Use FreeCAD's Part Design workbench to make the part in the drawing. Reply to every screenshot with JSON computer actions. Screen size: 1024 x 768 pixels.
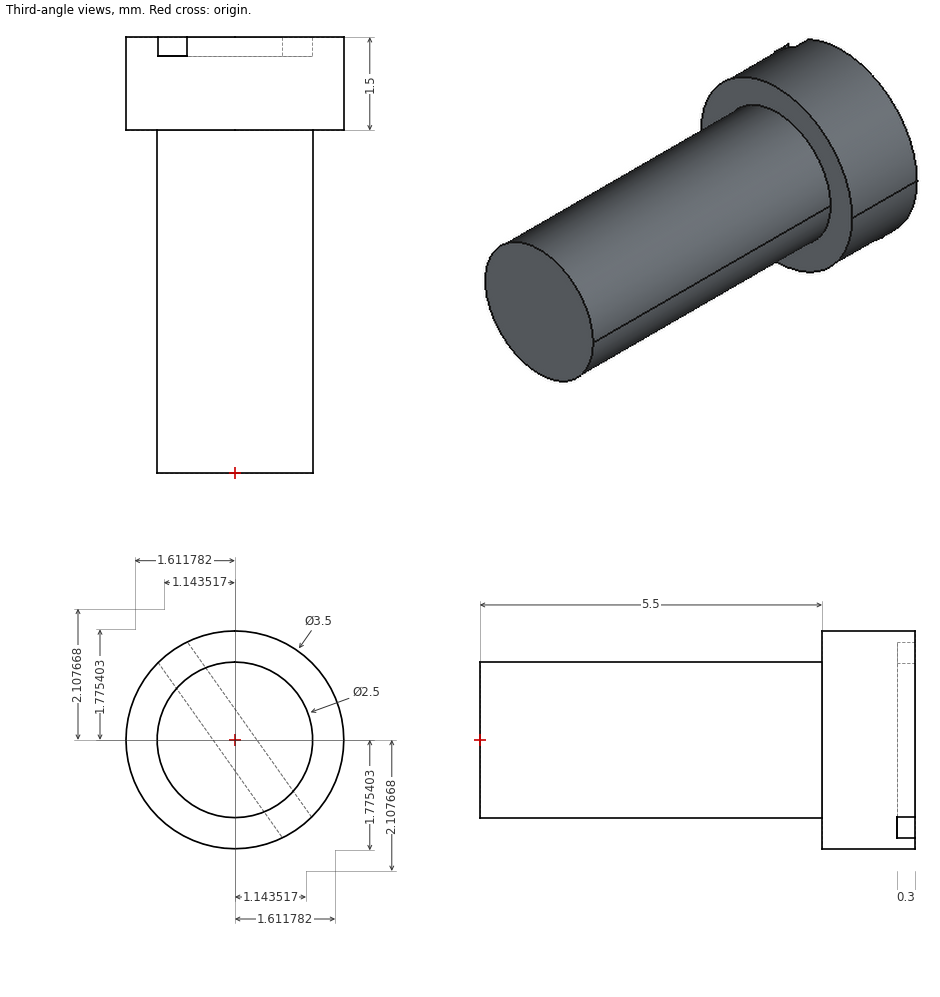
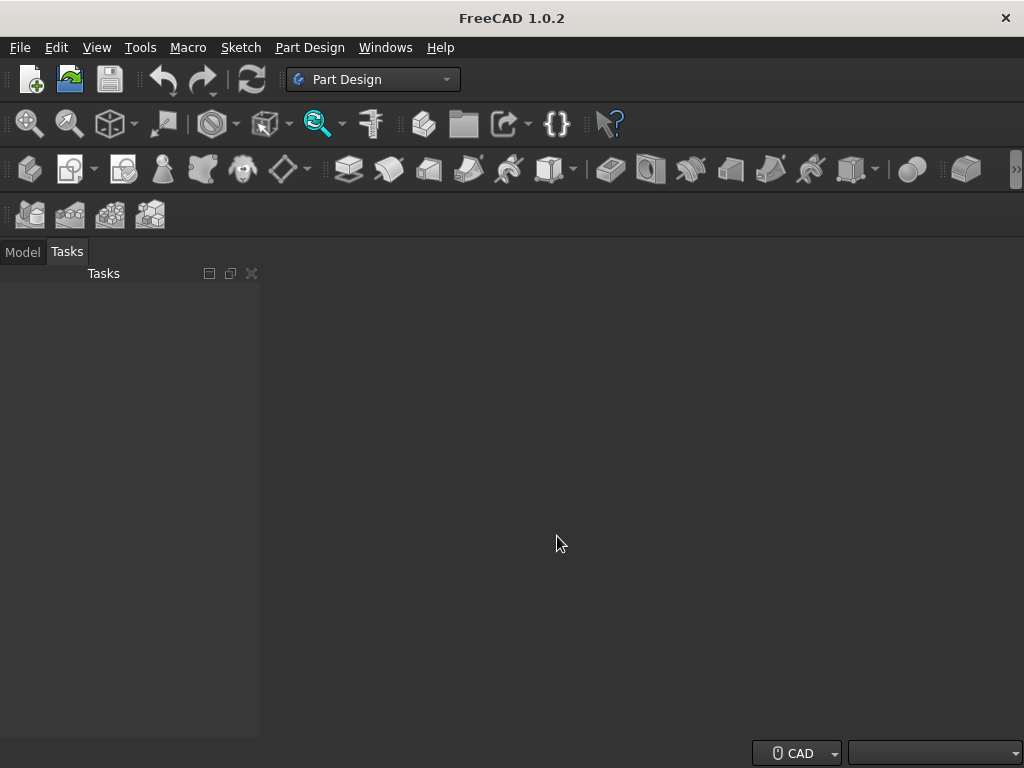
{"action": "key", "text": "ctrl+n"}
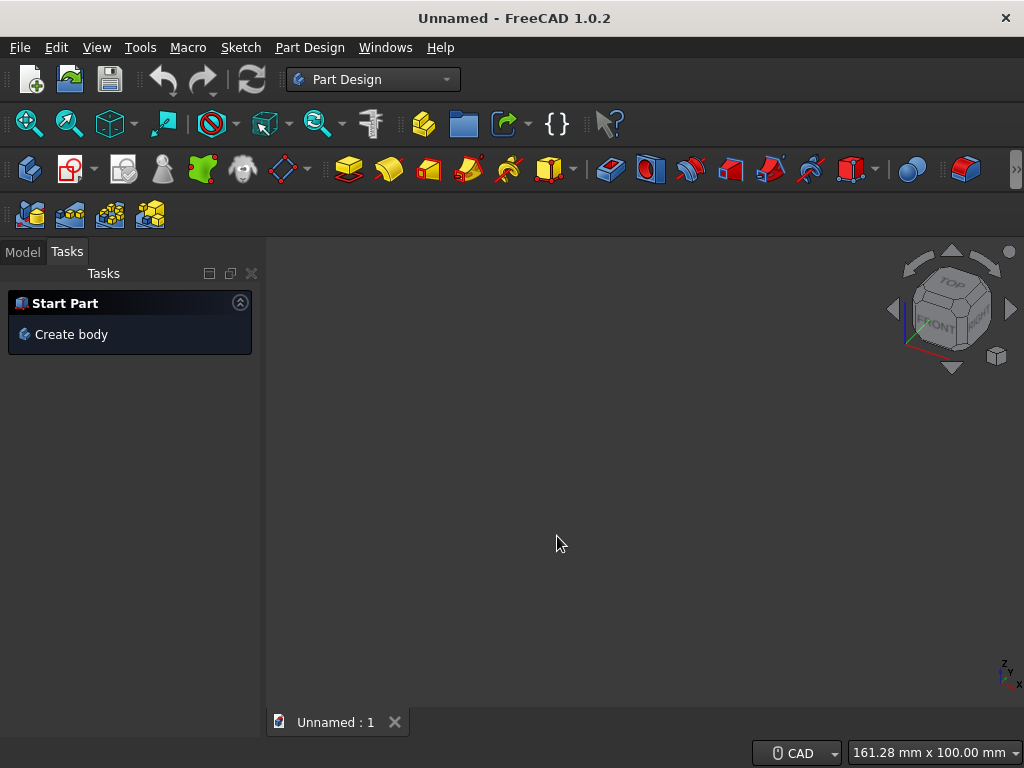
{"action": "left_click", "coordinate": [70, 170]}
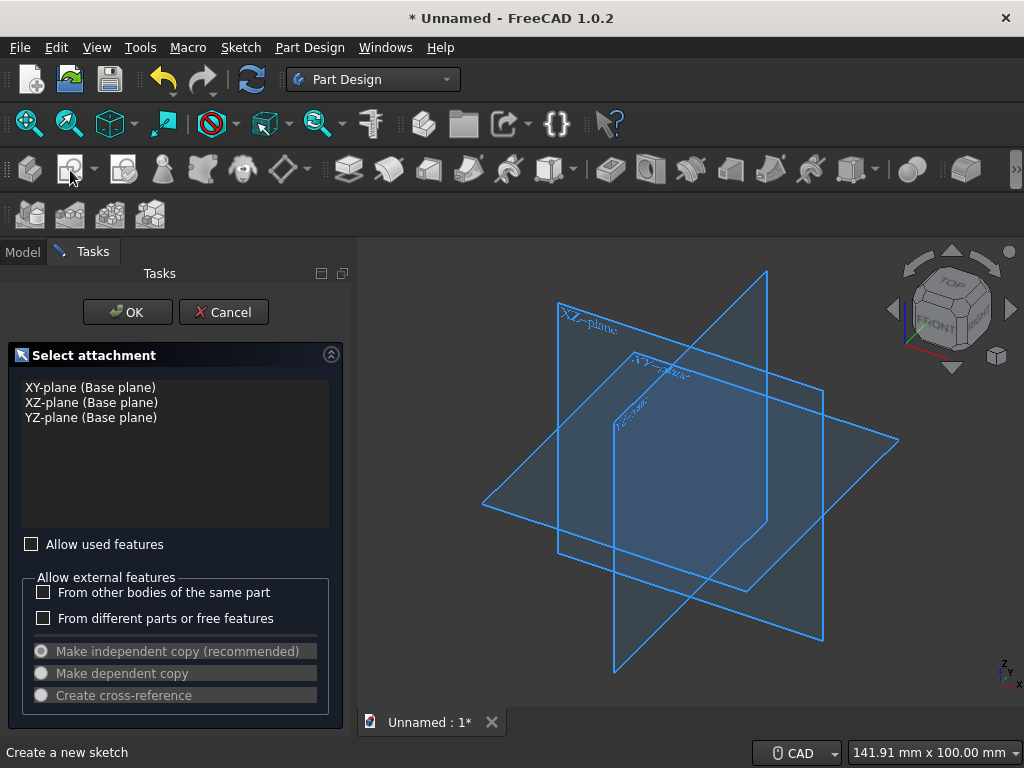
{"action": "left_click", "coordinate": [82, 402]}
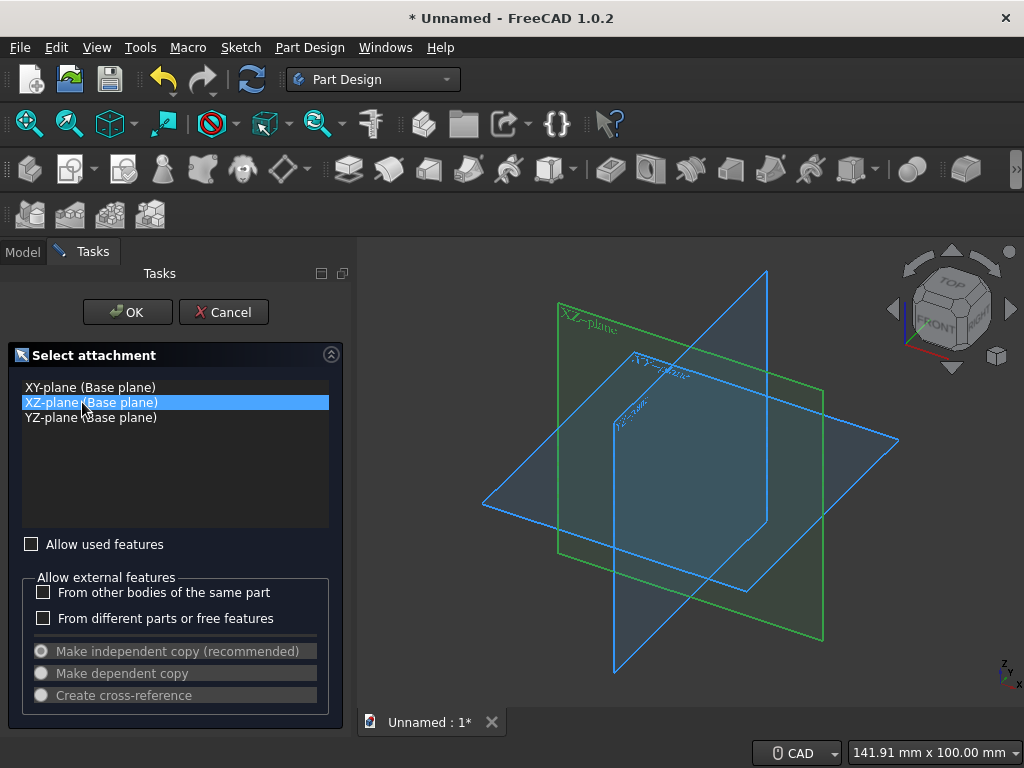
{"action": "left_click", "coordinate": [128, 312]}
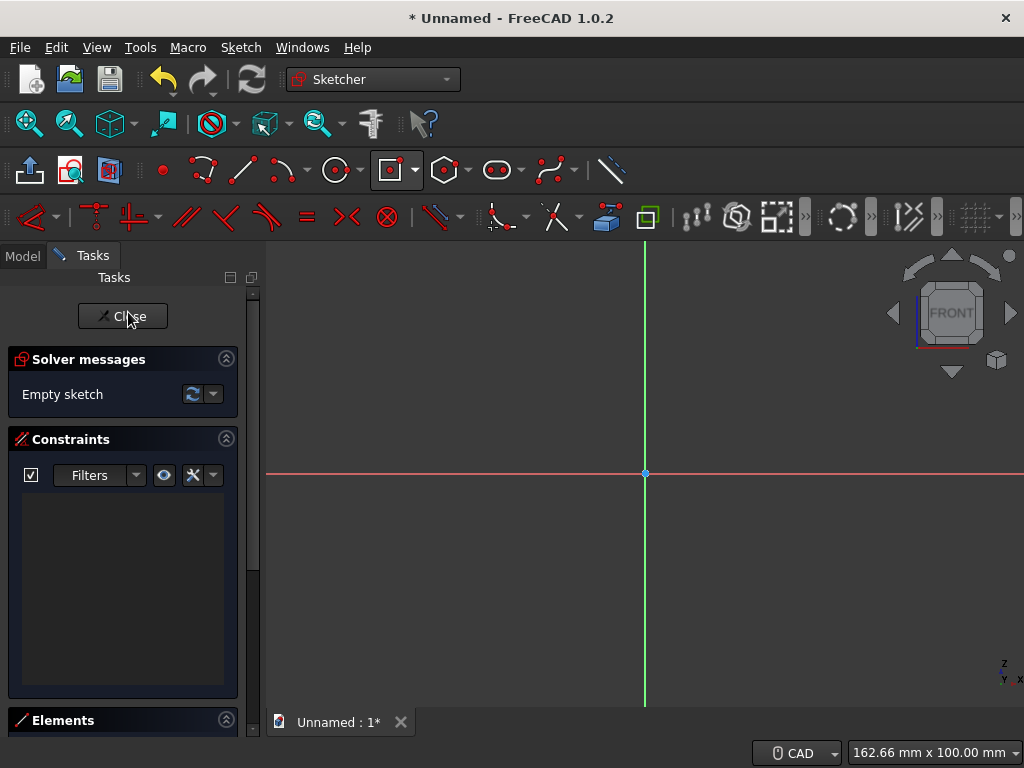
{"action": "scroll", "coordinate": [649, 474], "scroll_direction": "up", "scroll_amount": 15}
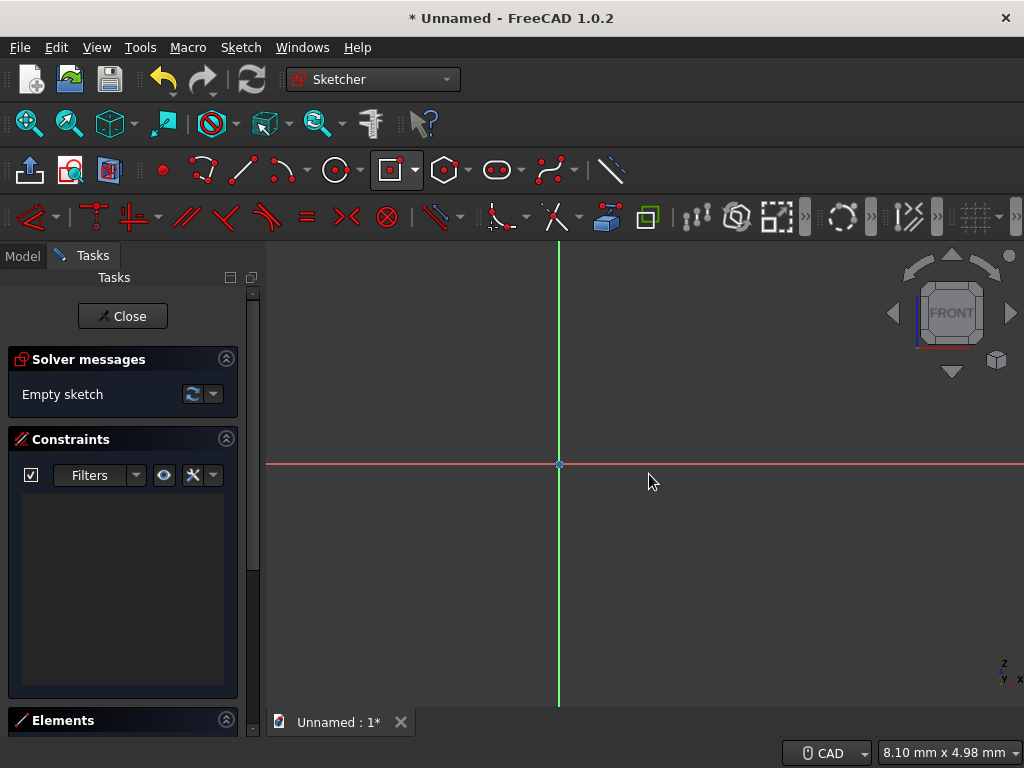
{"action": "key", "text": "g c"}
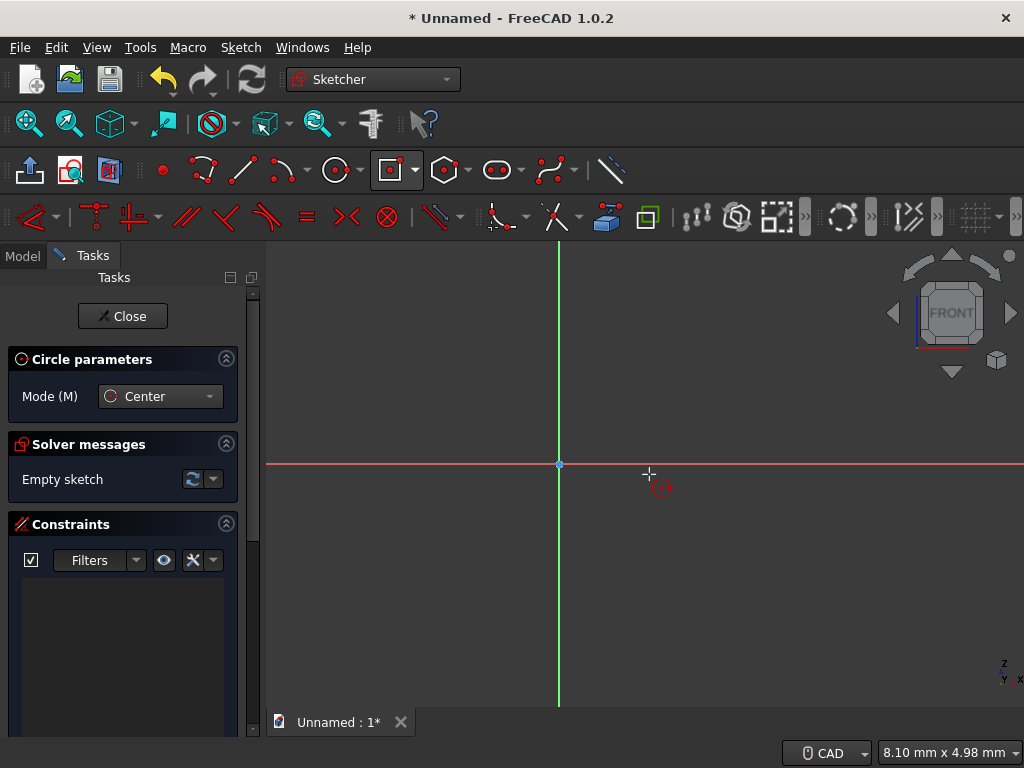
{"action": "left_click", "coordinate": [559, 464]}
{"action": "mouse_move", "coordinate": [642, 382]}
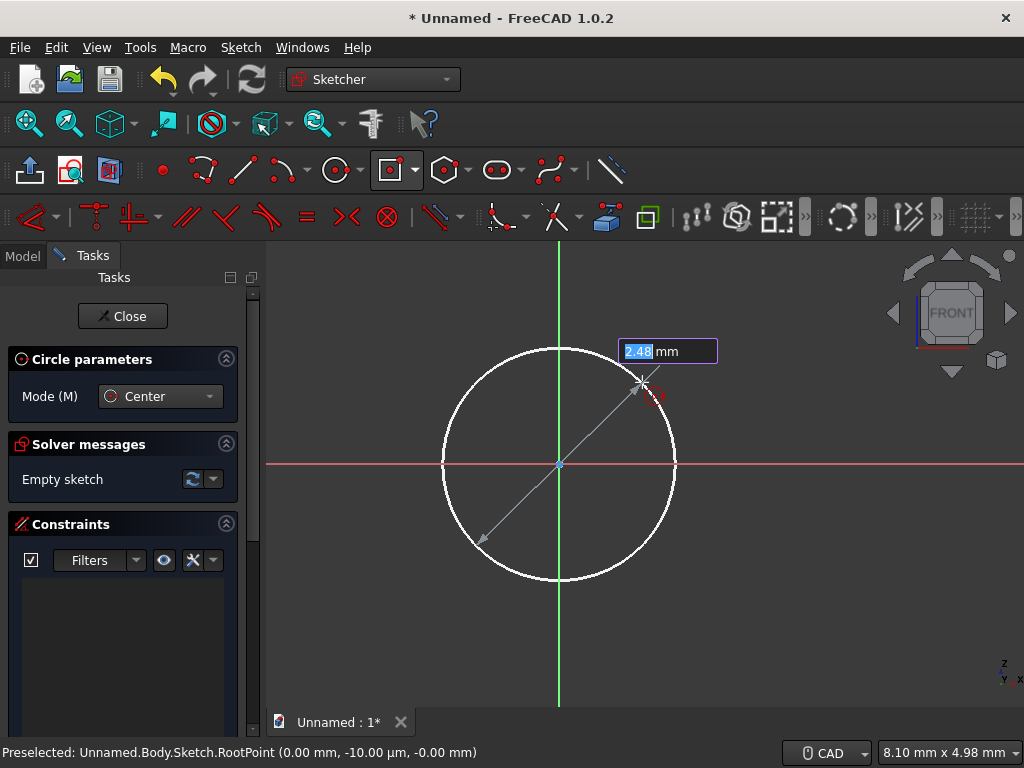
{"action": "type", "text": "2.5"}
{"action": "key", "text": "Return"}
{"action": "key", "text": "Escape"}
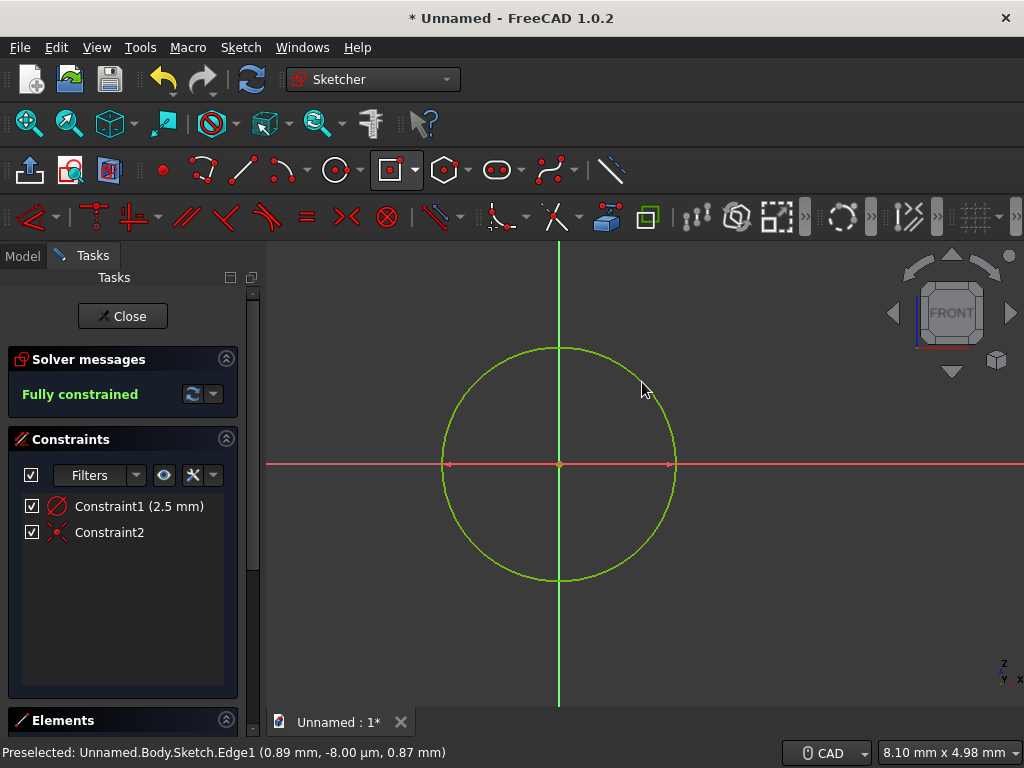
{"action": "left_click", "coordinate": [123, 316]}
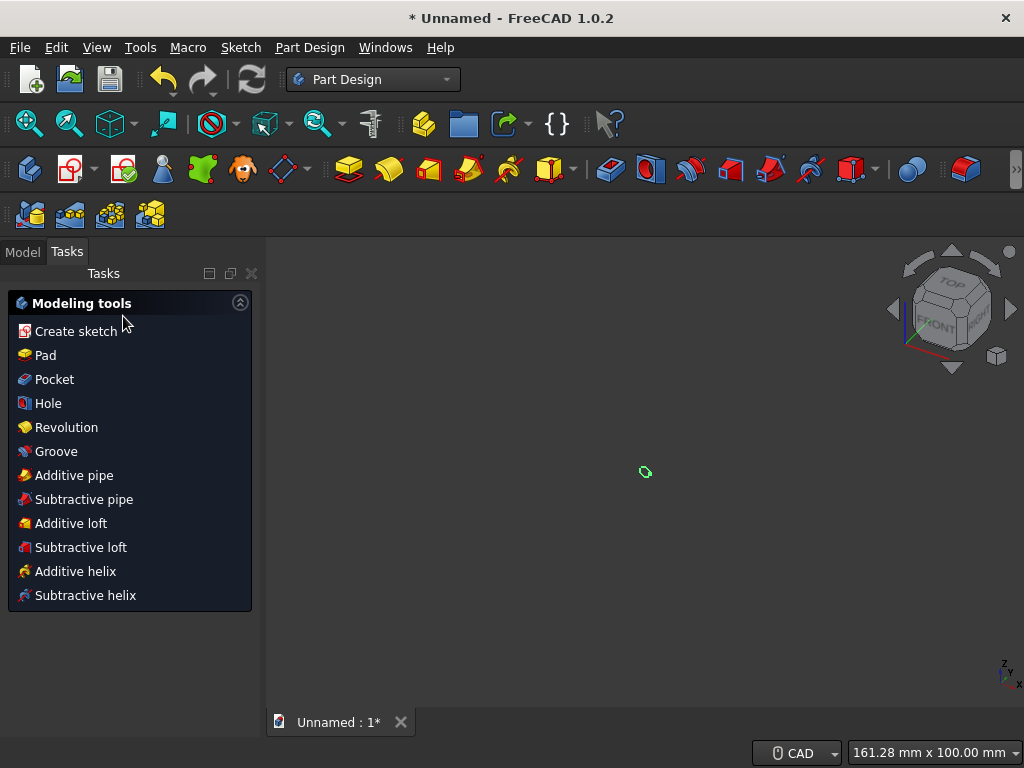
{"action": "left_click", "coordinate": [350, 170]}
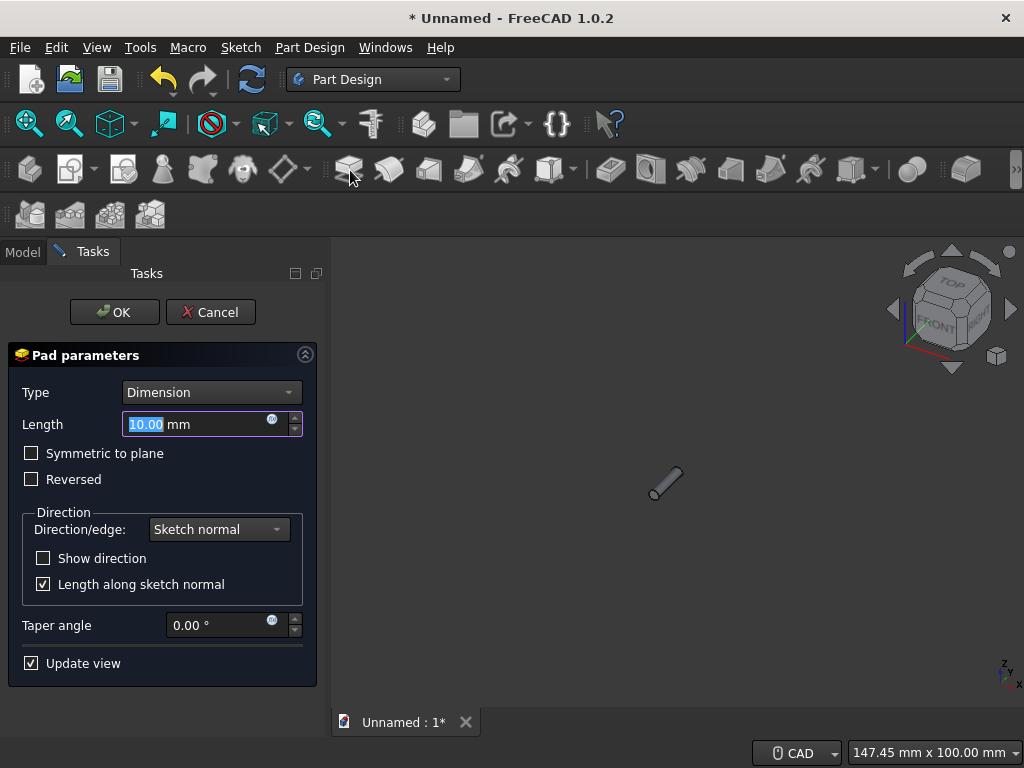
{"action": "type", "text": "5.5"}
{"action": "key", "text": "Tab"}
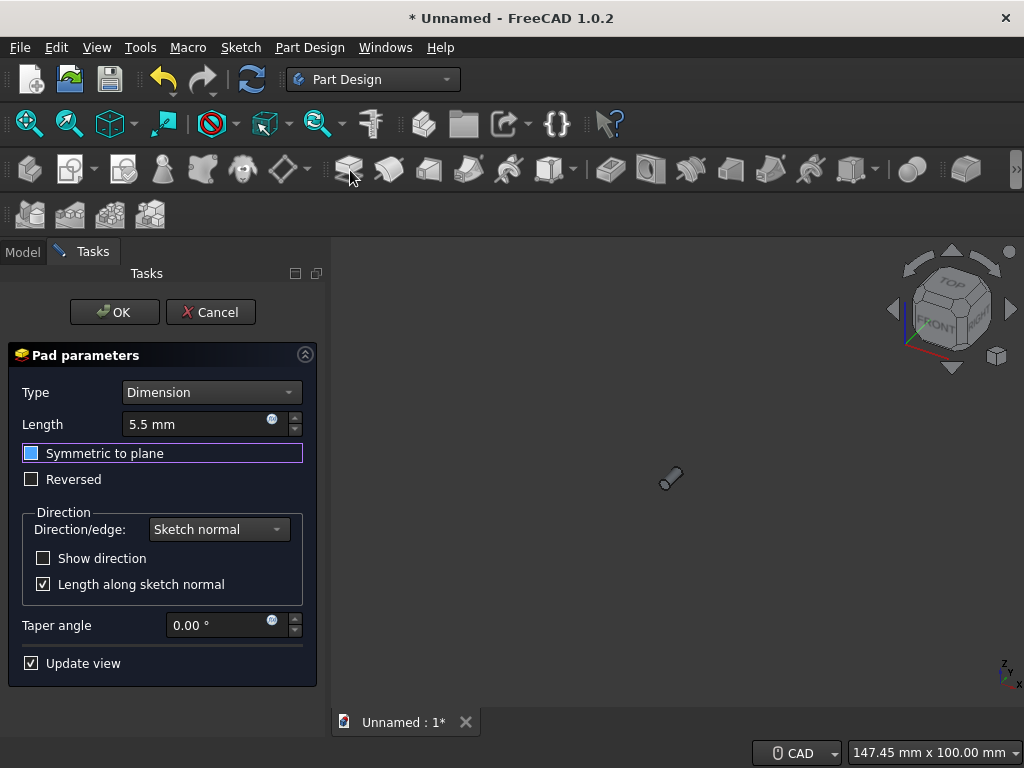
{"action": "left_click", "coordinate": [30, 479]}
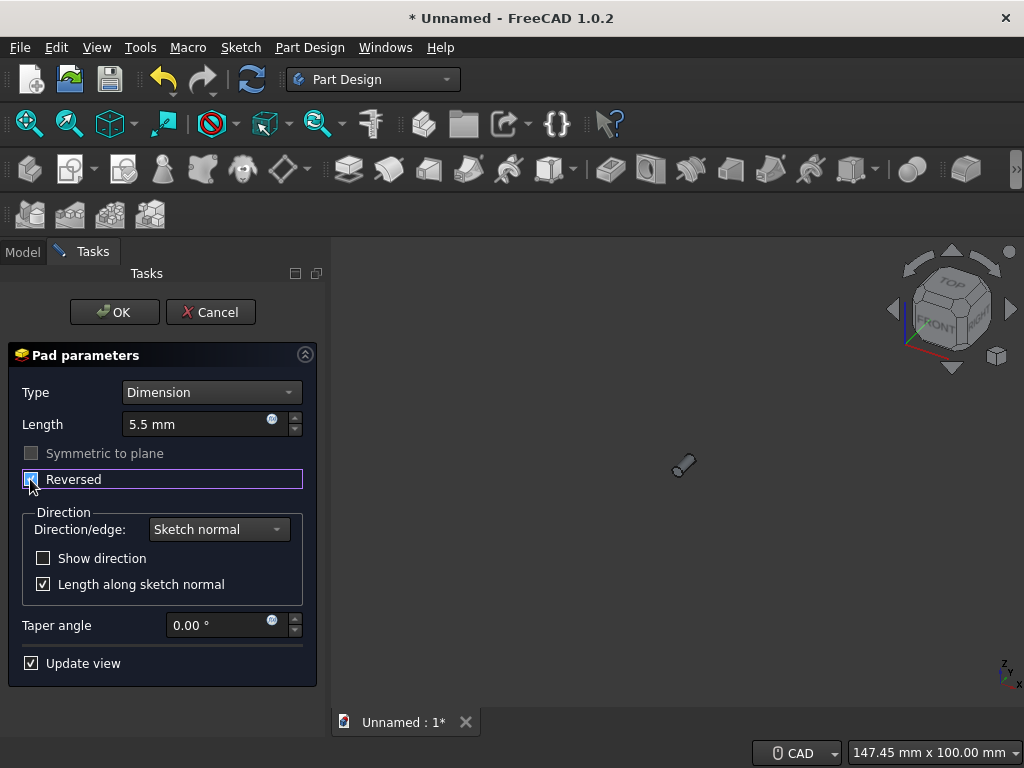
{"action": "left_click", "coordinate": [115, 312]}